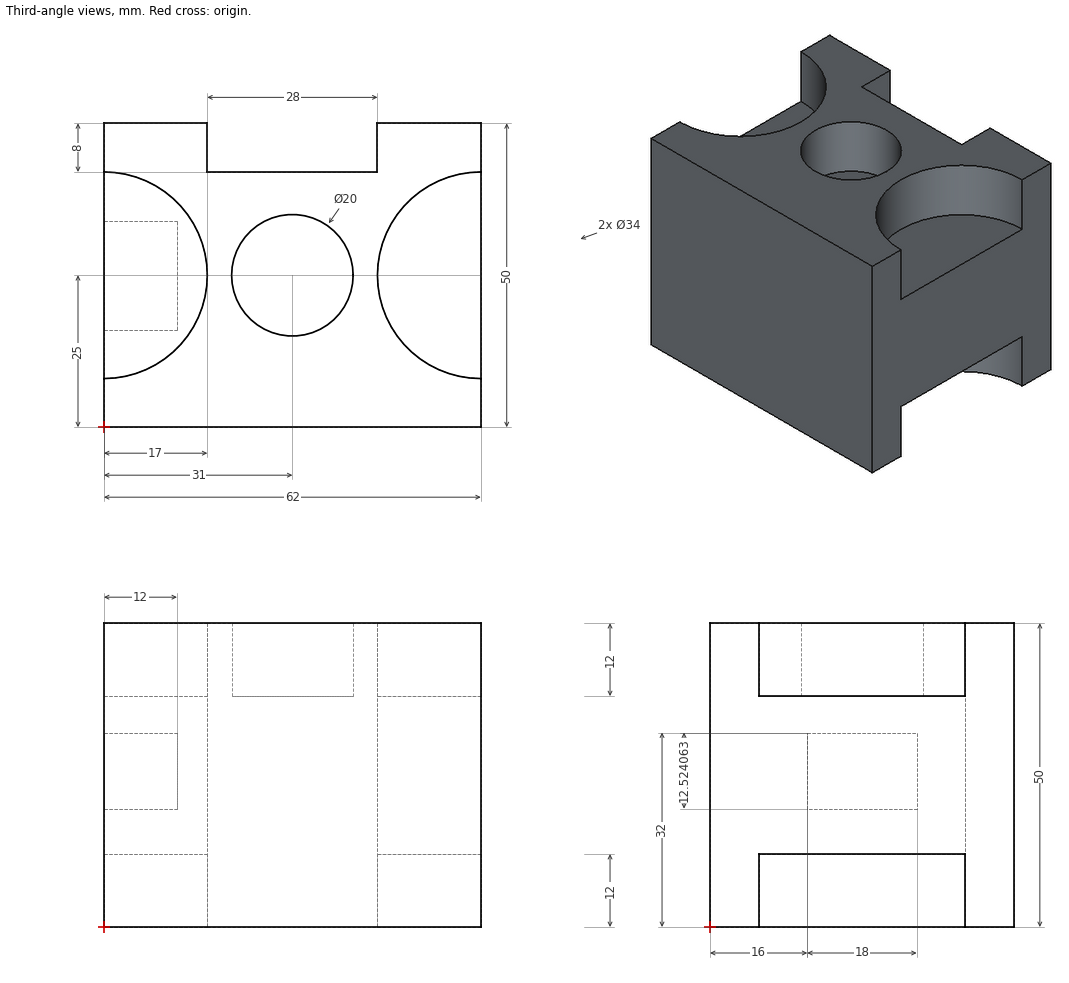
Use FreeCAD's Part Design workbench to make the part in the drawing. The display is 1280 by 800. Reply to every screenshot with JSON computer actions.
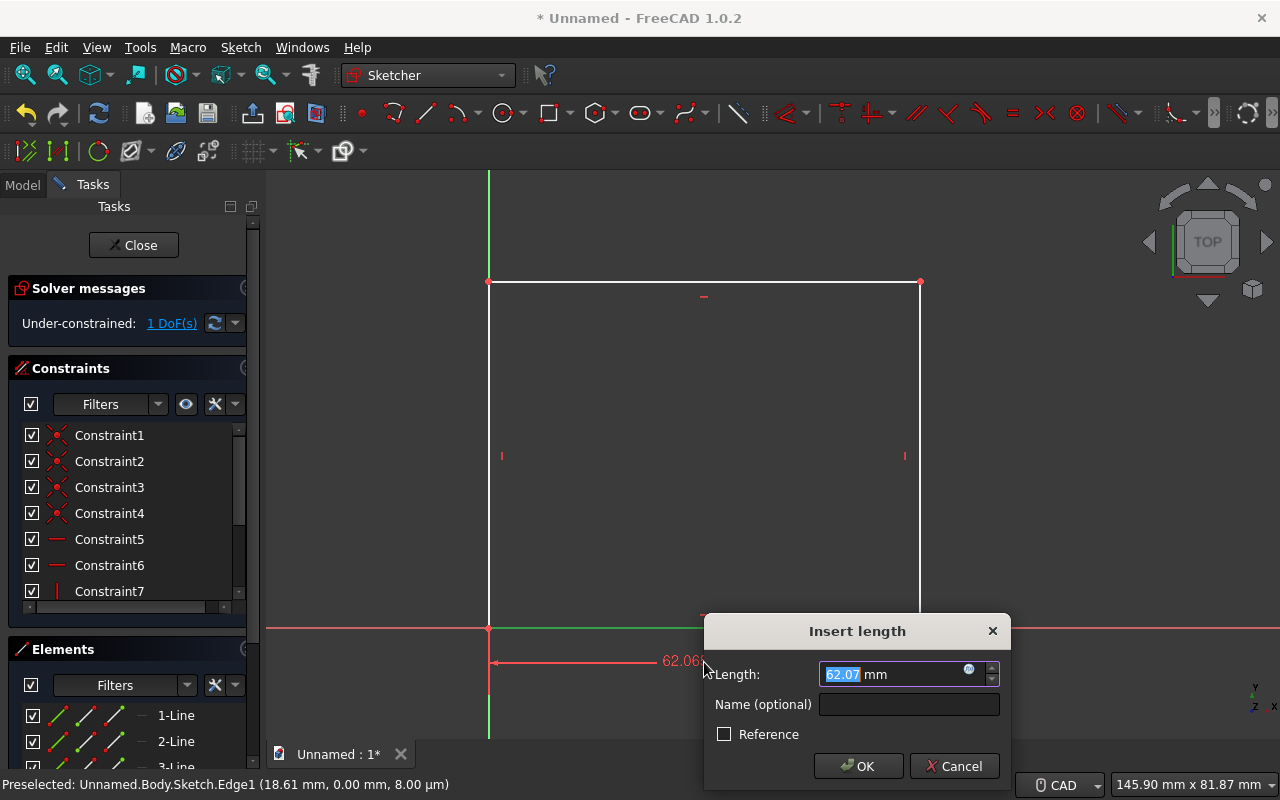
{"action": "type", "text": "62"}
{"action": "key", "text": "Return"}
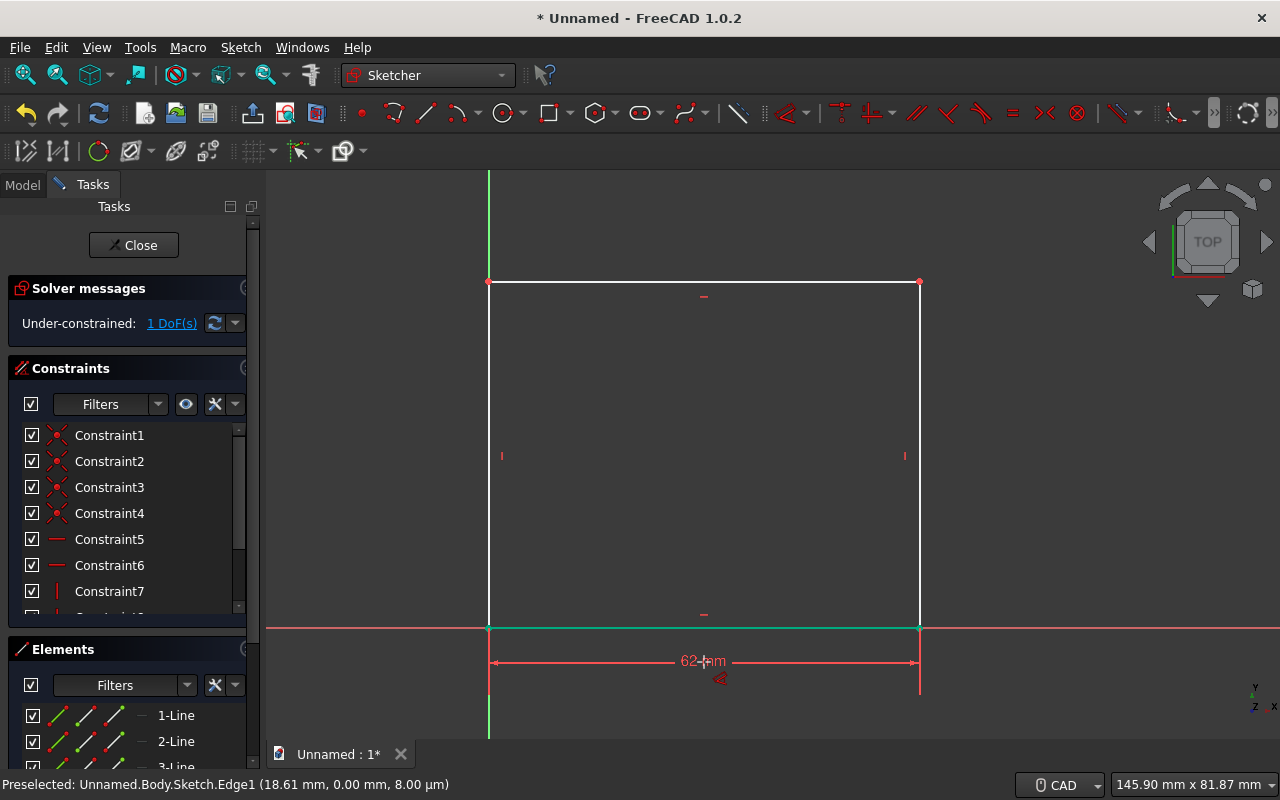
{"action": "left_click", "coordinate": [920, 524]}
{"action": "left_click", "coordinate": [954, 455]}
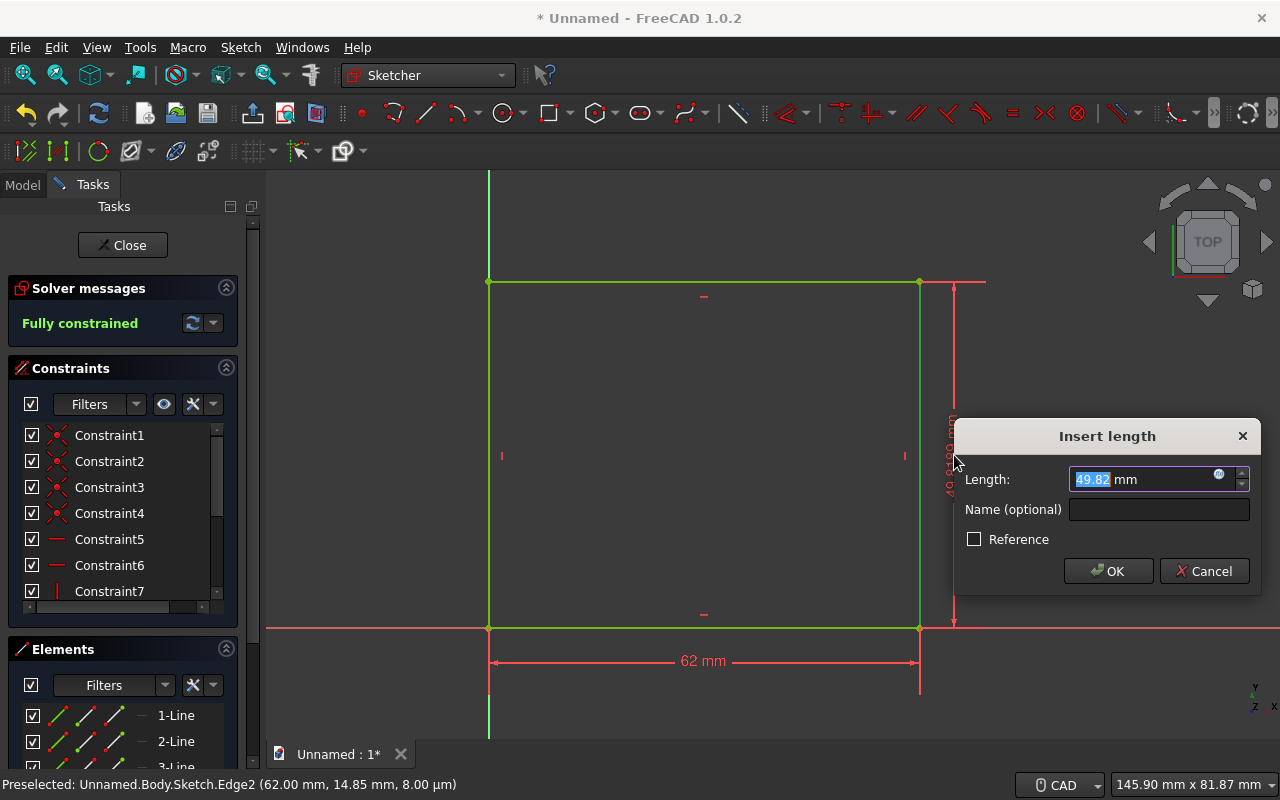
{"action": "type", "text": "50"}
{"action": "key", "text": "Return"}
{"action": "key", "text": "Escape"}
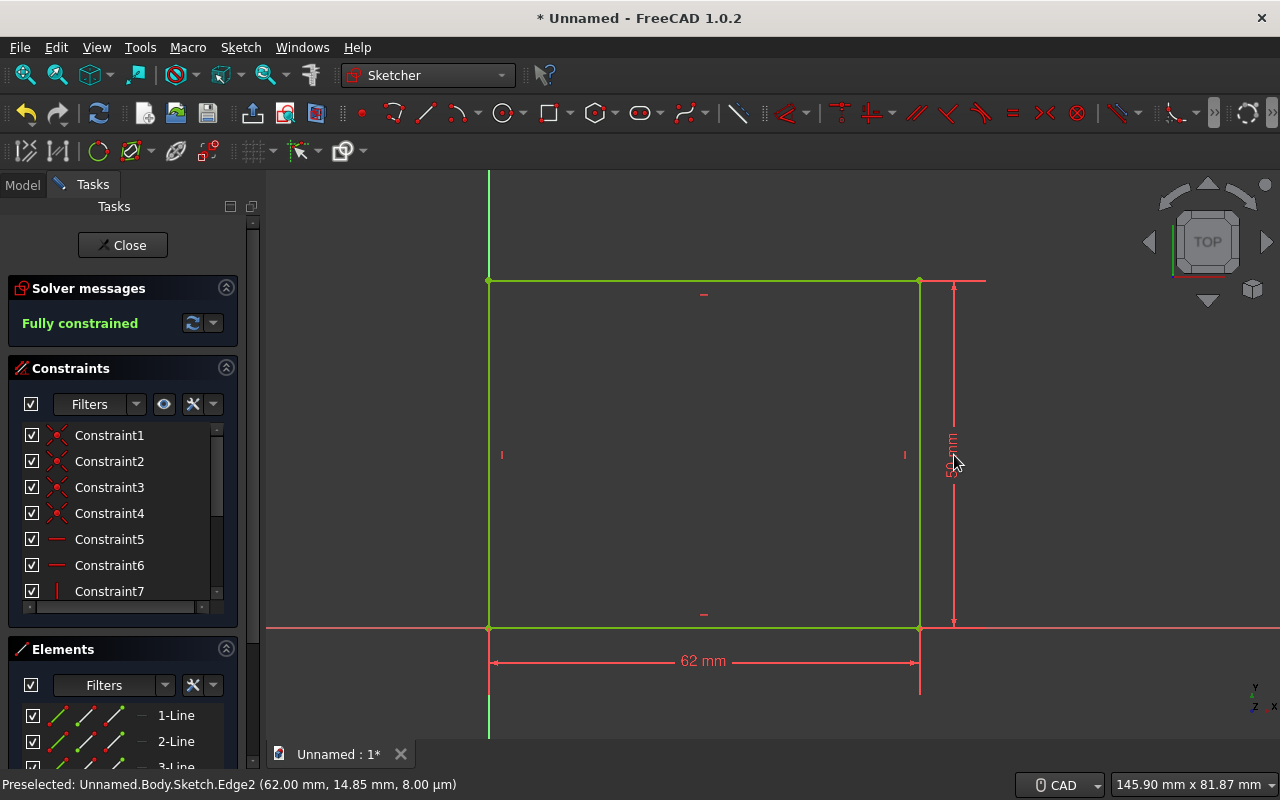
{"action": "left_click", "coordinate": [123, 245]}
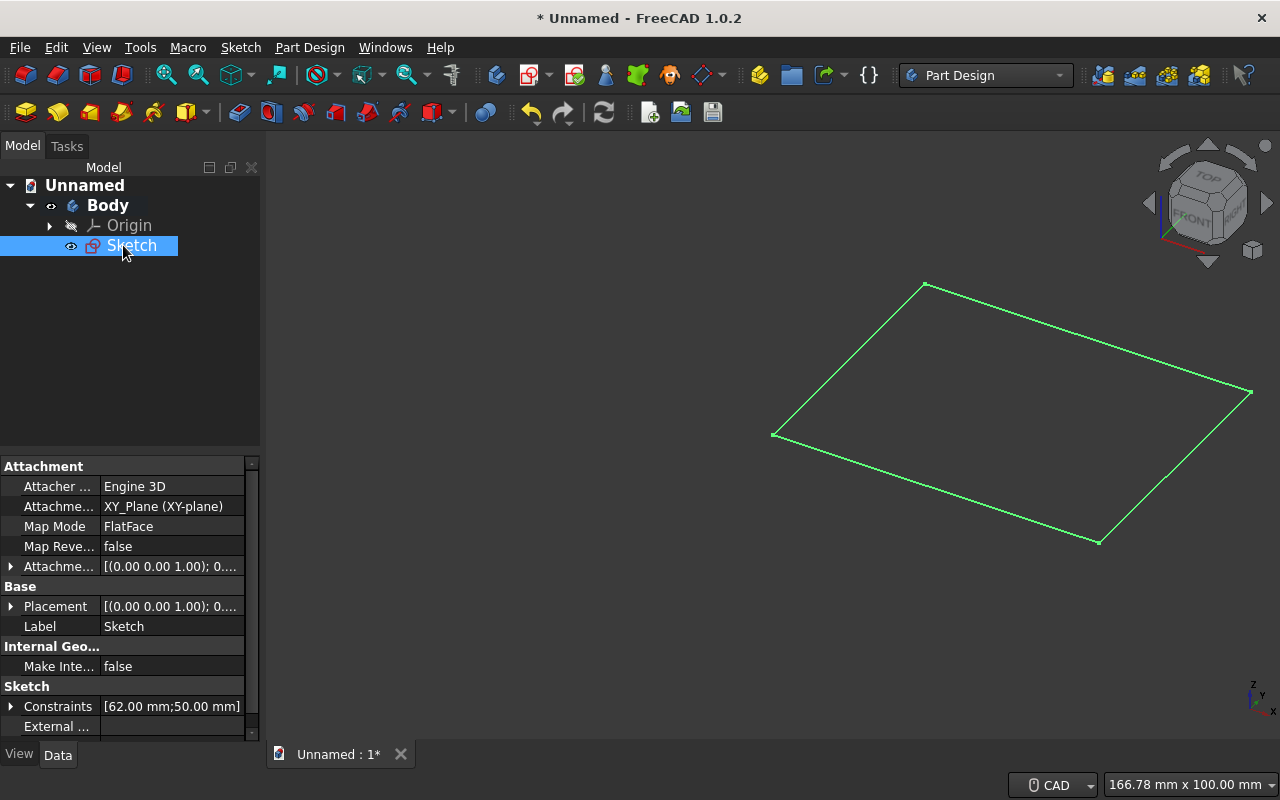
{"action": "left_click", "coordinate": [26, 112]}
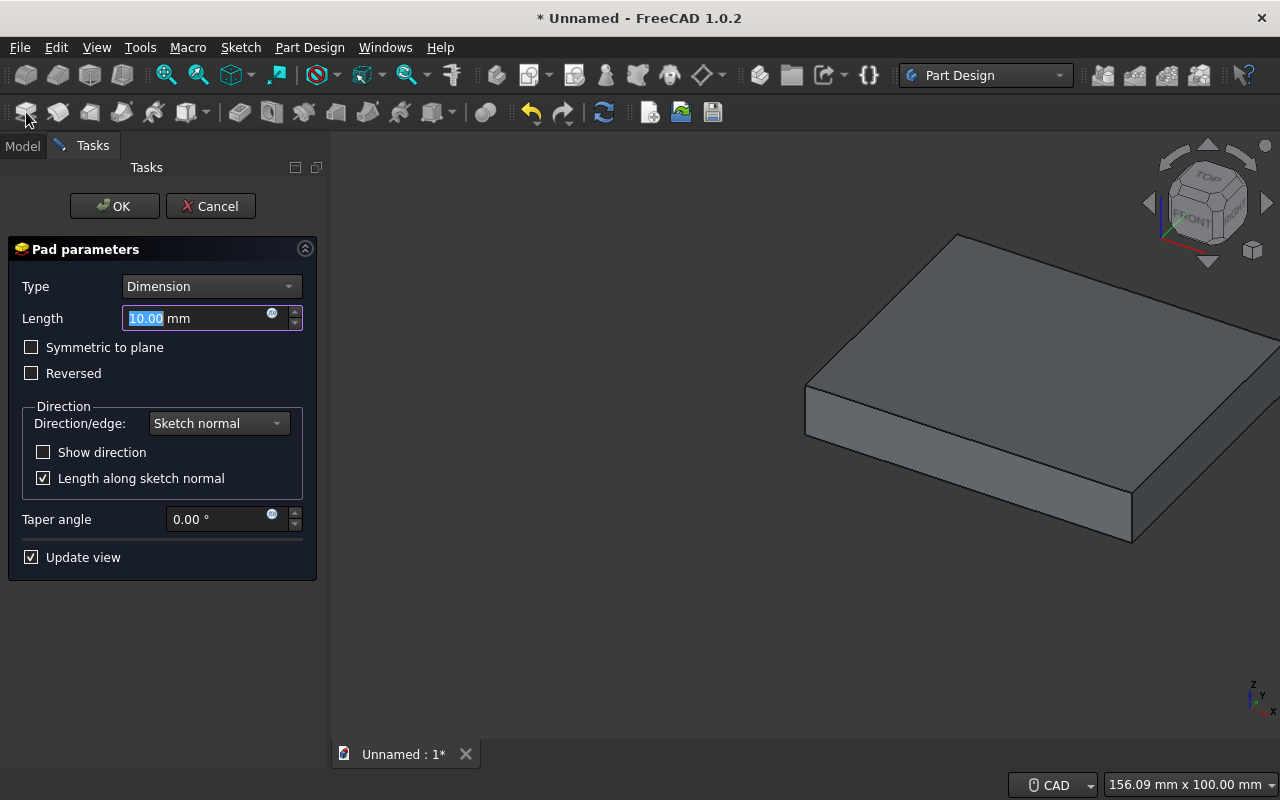
{"action": "type", "text": "50"}
{"action": "key", "text": "Tab"}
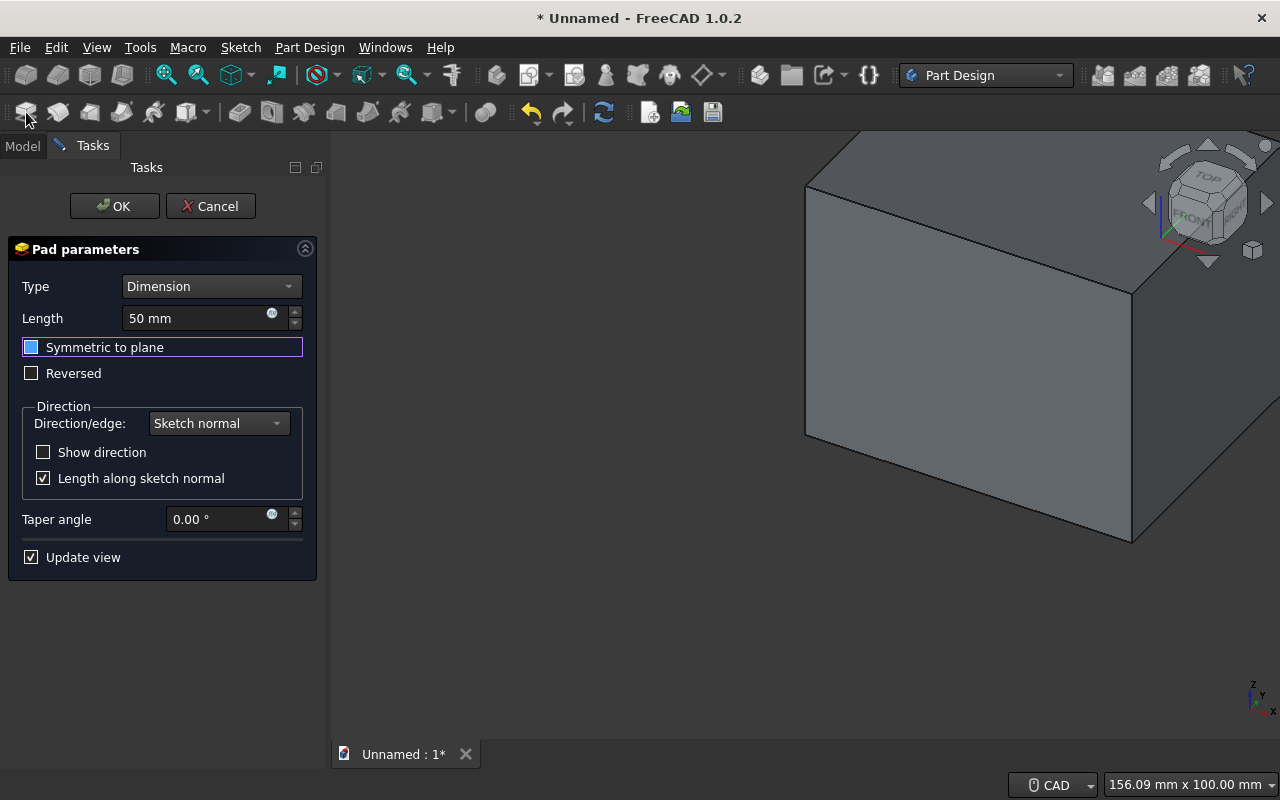
{"action": "left_click", "coordinate": [115, 206]}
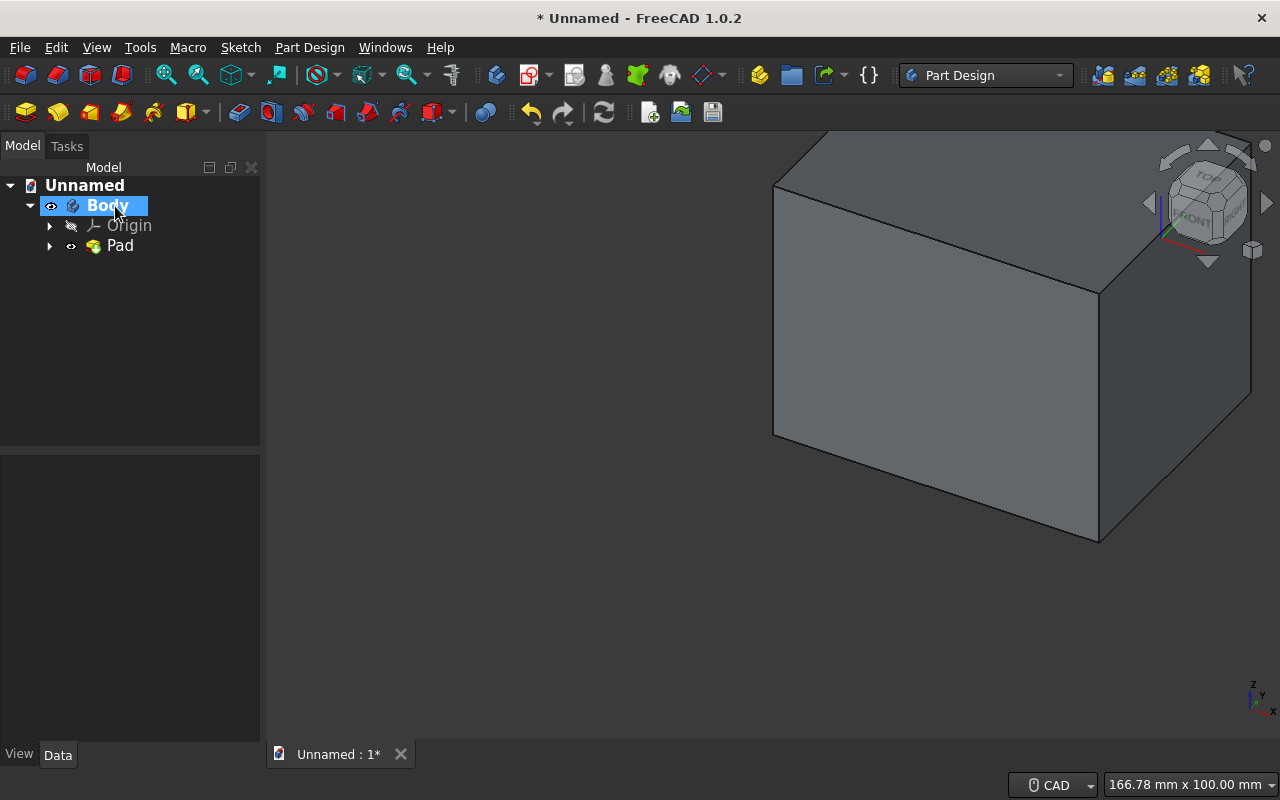
{"action": "left_click", "coordinate": [168, 76]}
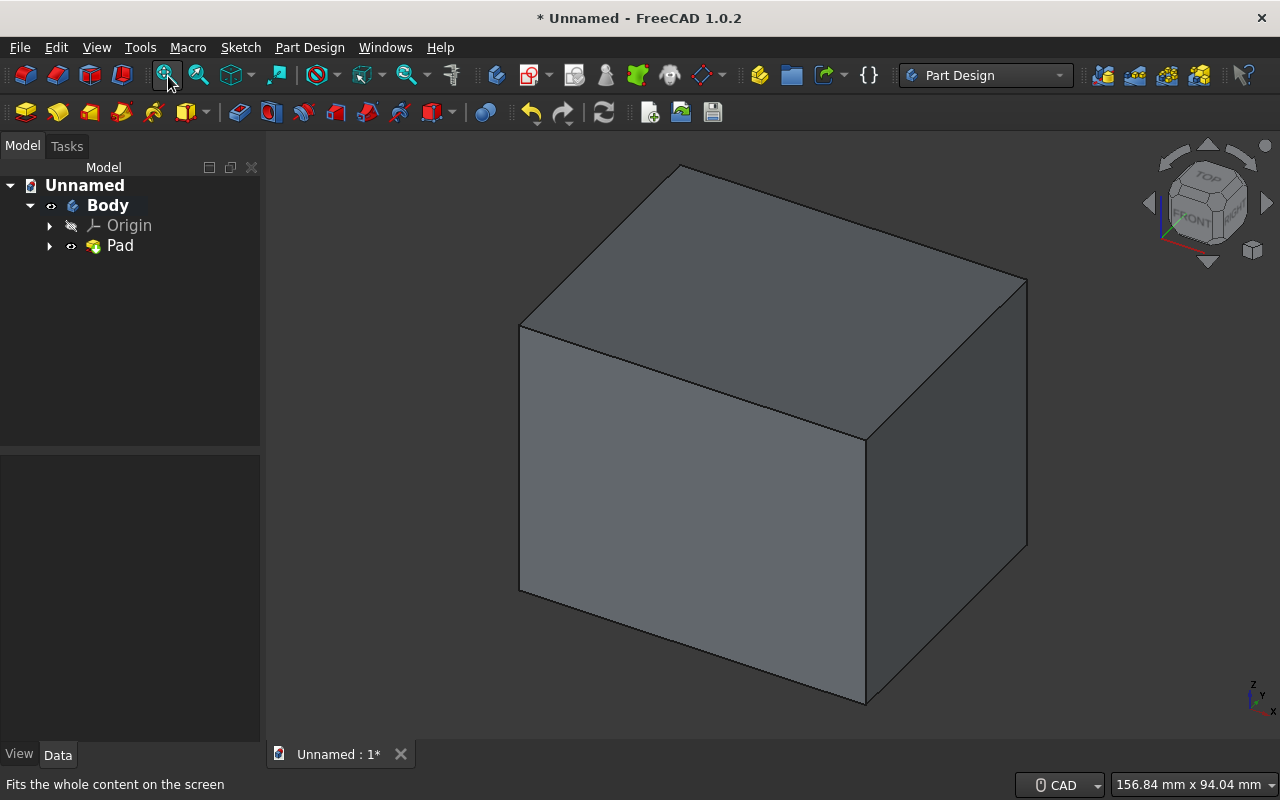
{"action": "left_click", "coordinate": [773, 302]}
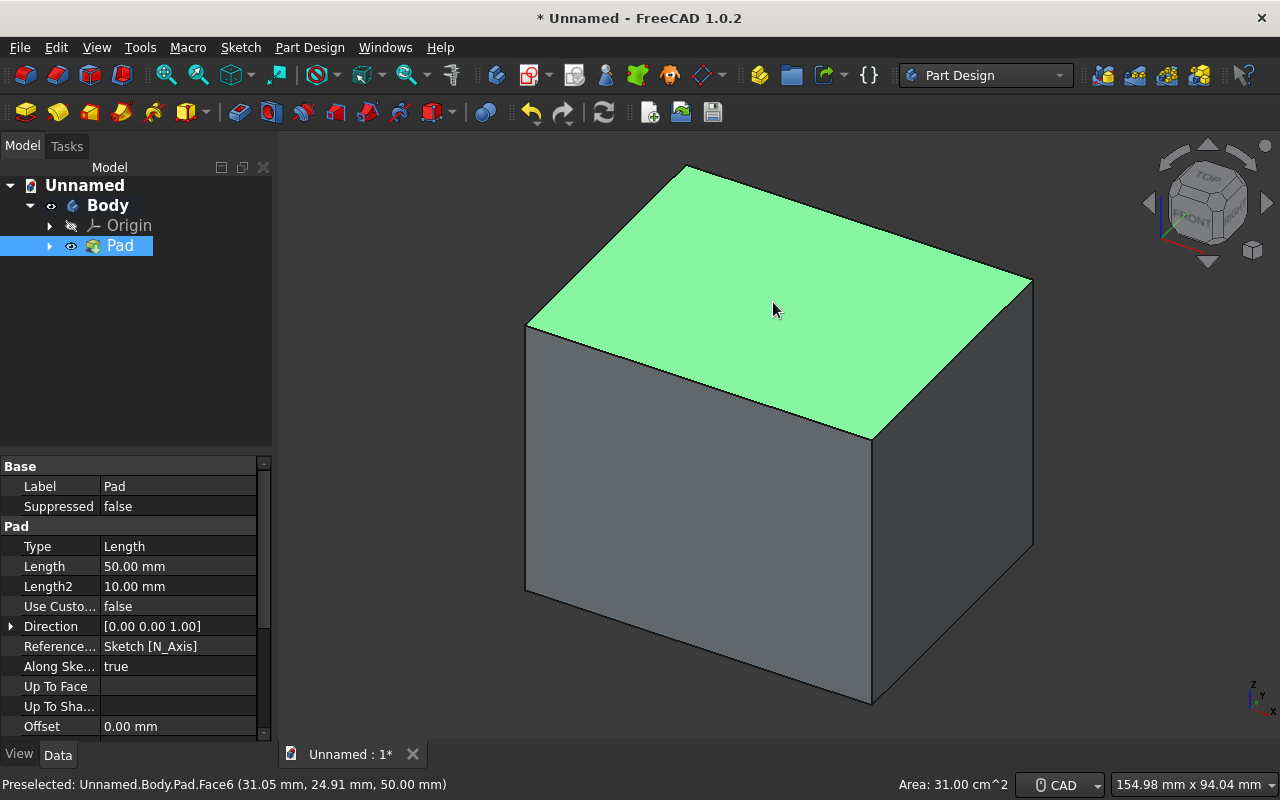
{"action": "left_click", "coordinate": [530, 76]}